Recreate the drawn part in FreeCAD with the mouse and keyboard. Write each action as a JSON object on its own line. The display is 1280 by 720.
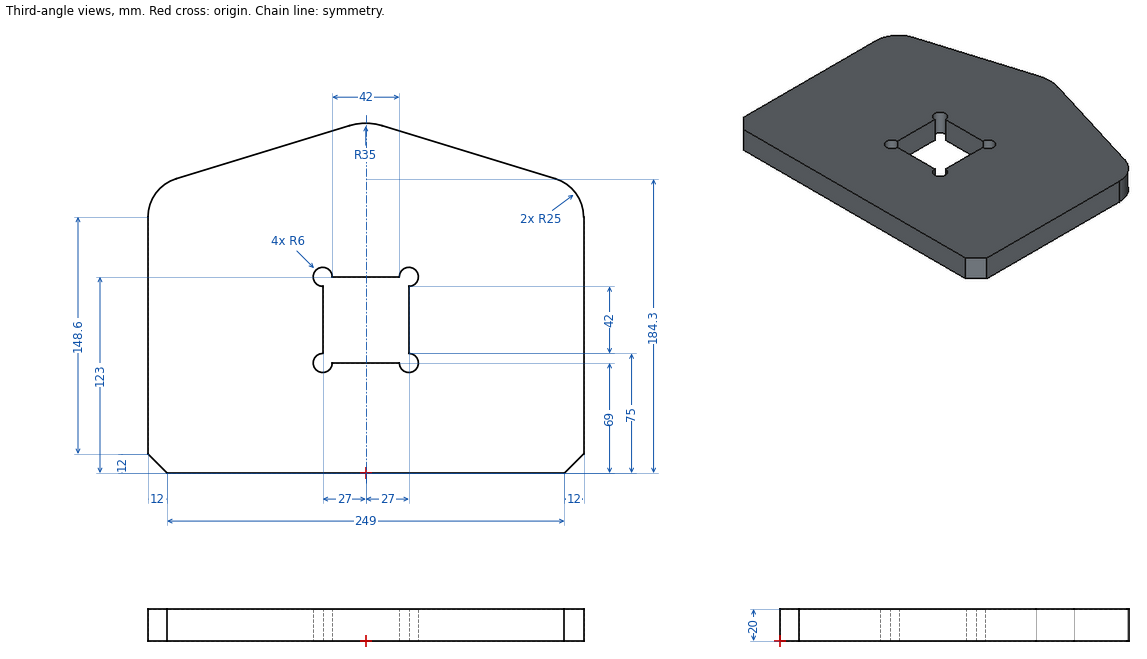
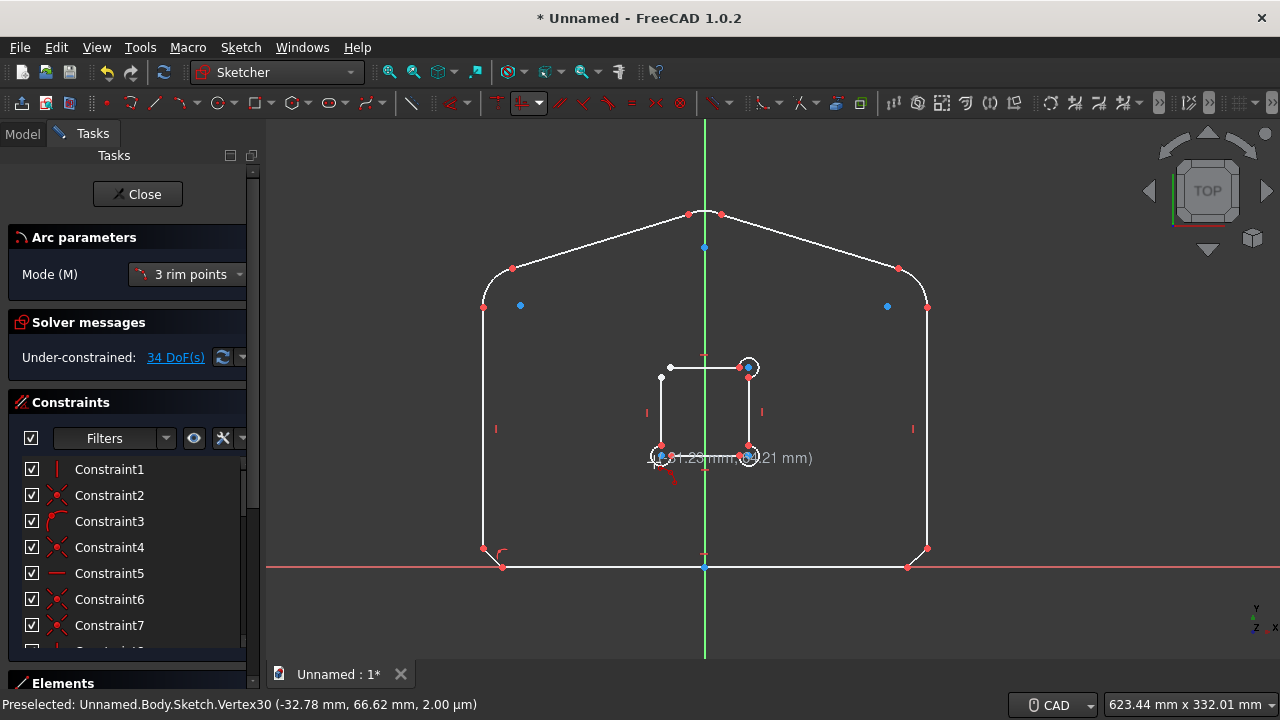
{"action": "left_click", "coordinate": [661, 378]}
{"action": "left_click", "coordinate": [670, 368]}
{"action": "left_click", "coordinate": [654, 360]}
{"action": "key", "text": "Escape"}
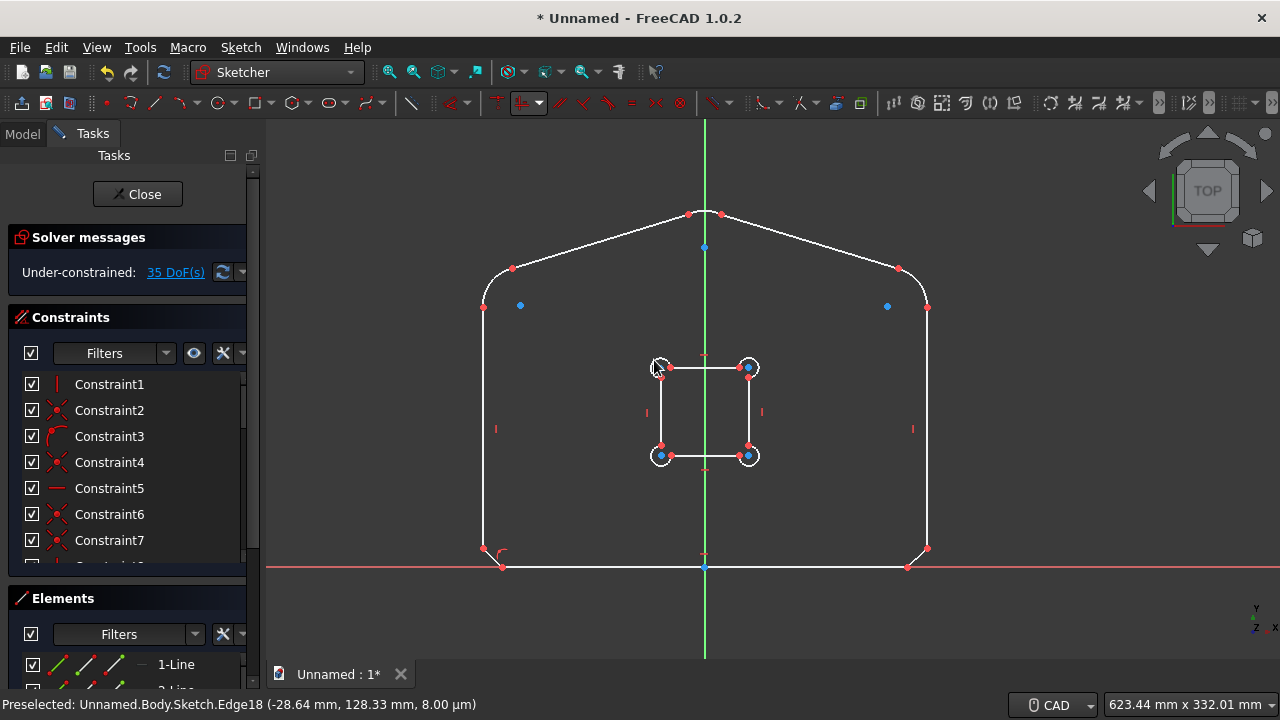
{"action": "left_click", "coordinate": [845, 252]}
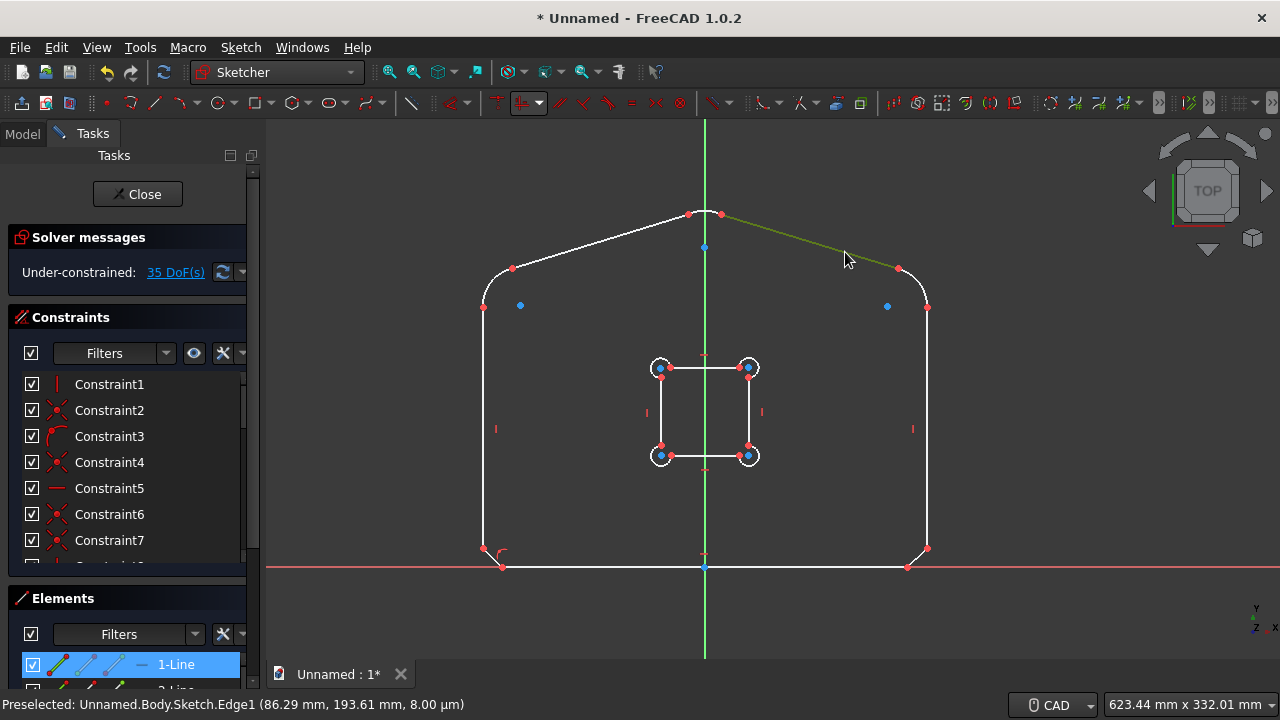
{"action": "left_click", "coordinate": [704, 211]}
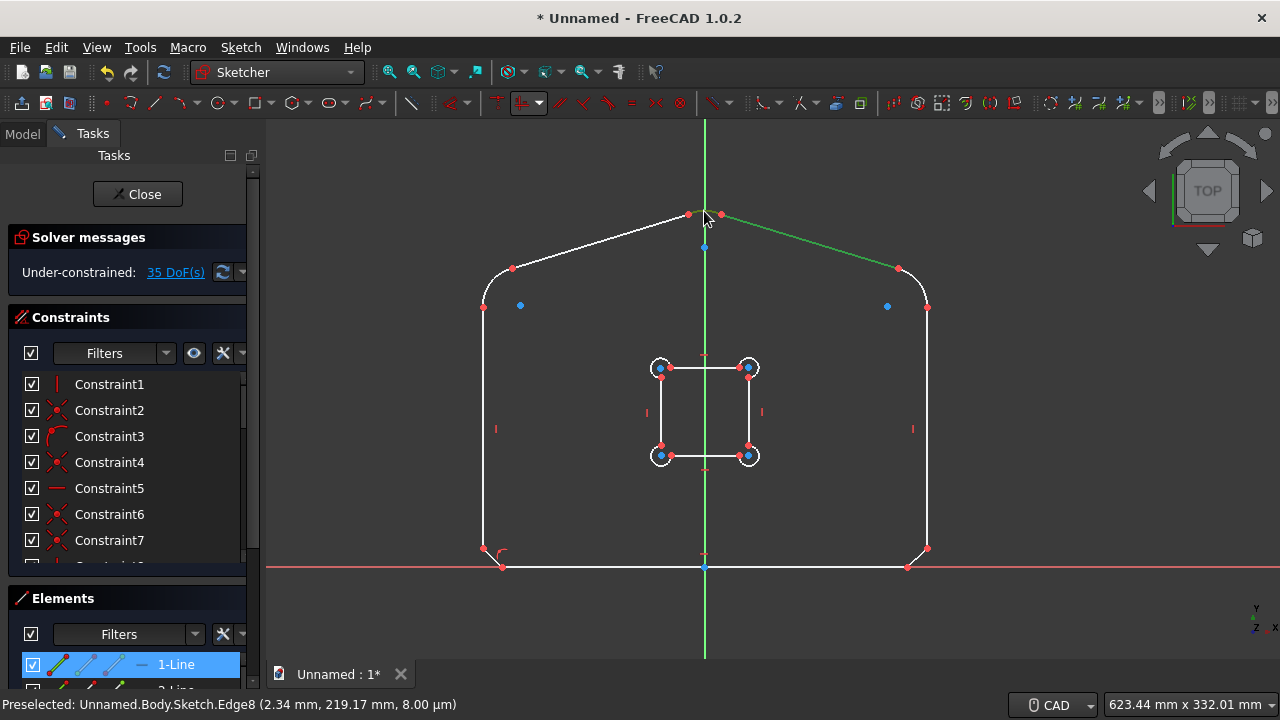
{"action": "left_click", "coordinate": [608, 104]}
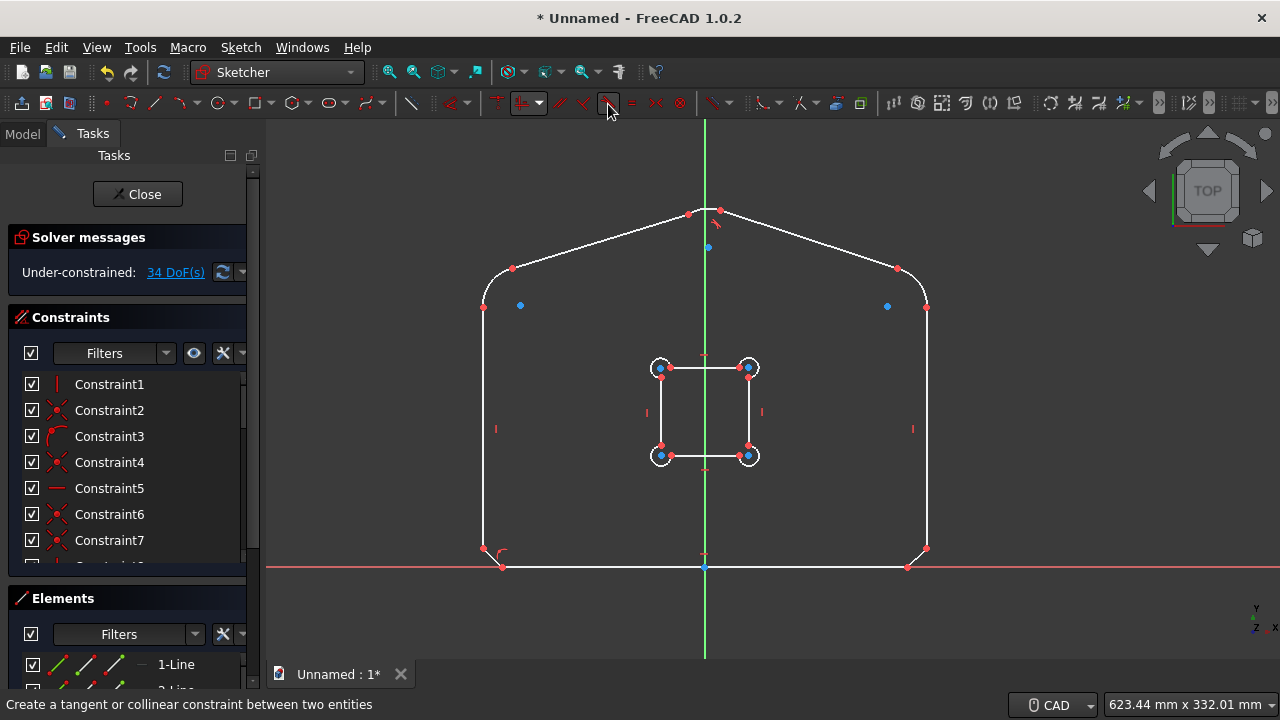
{"action": "left_click", "coordinate": [845, 251]}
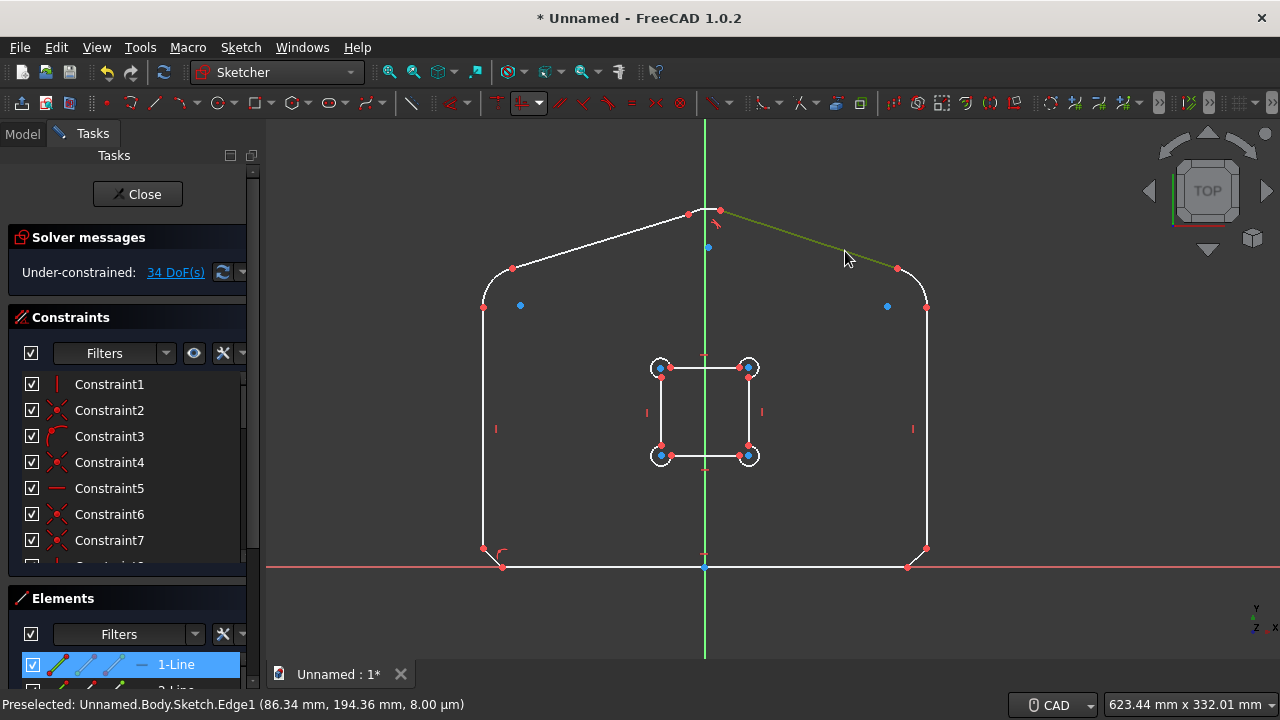
{"action": "left_click", "coordinate": [924, 292]}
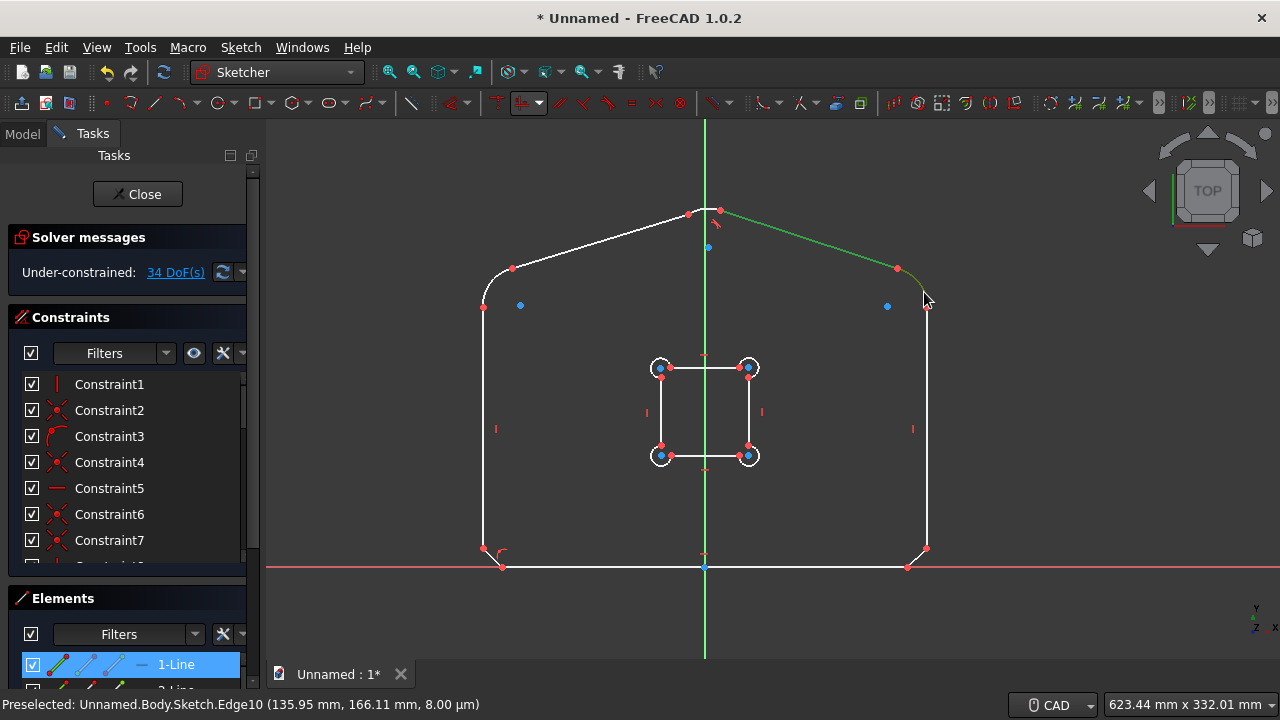
{"action": "left_click", "coordinate": [608, 104]}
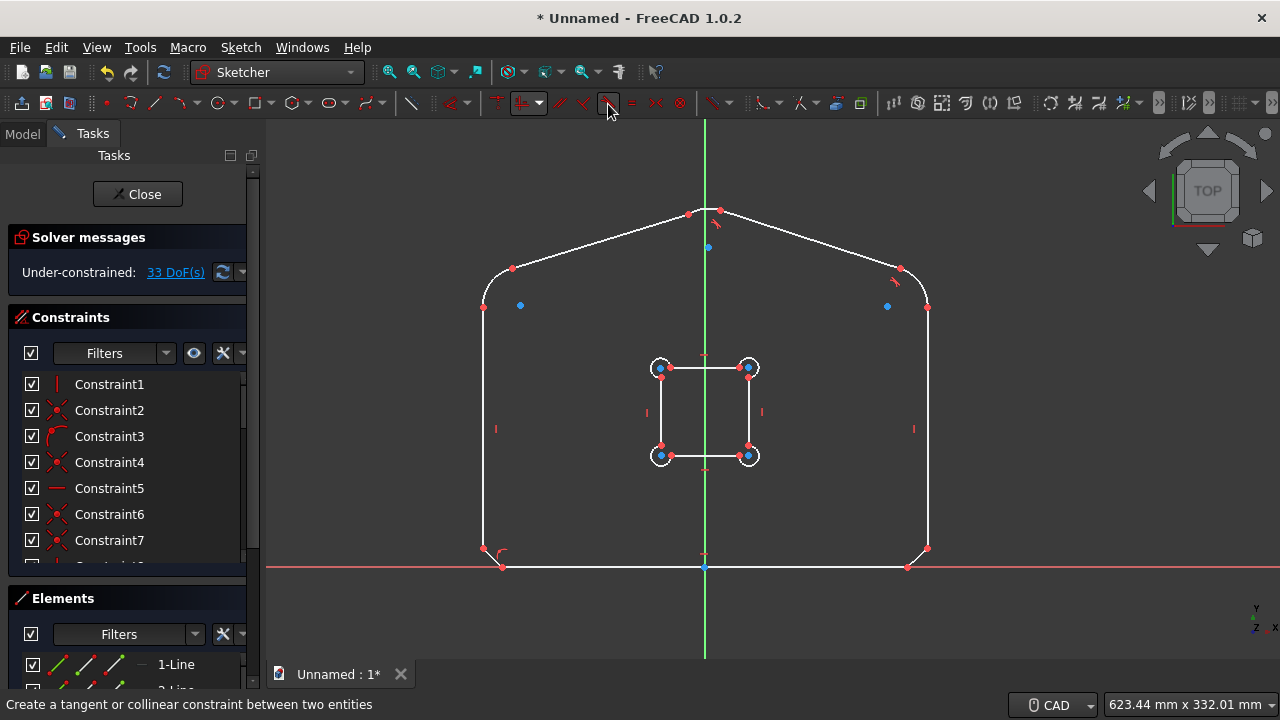
{"action": "left_click", "coordinate": [635, 231]}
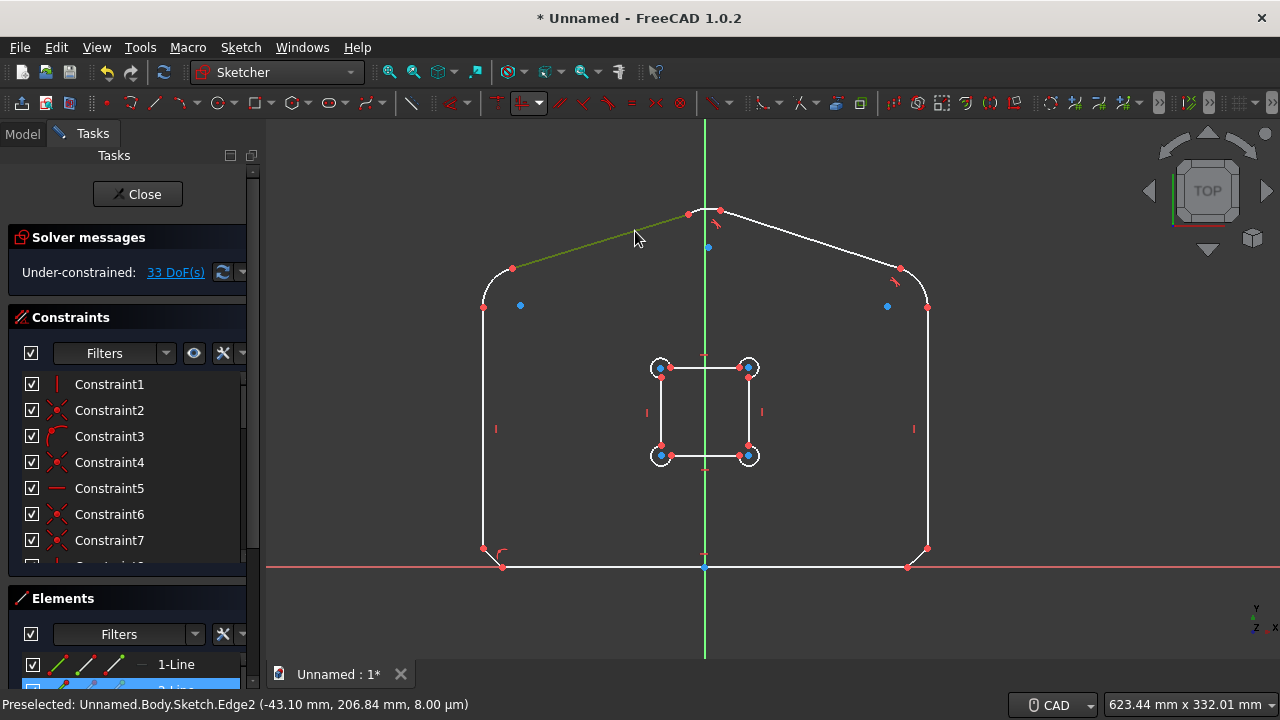
{"action": "left_click", "coordinate": [704, 209]}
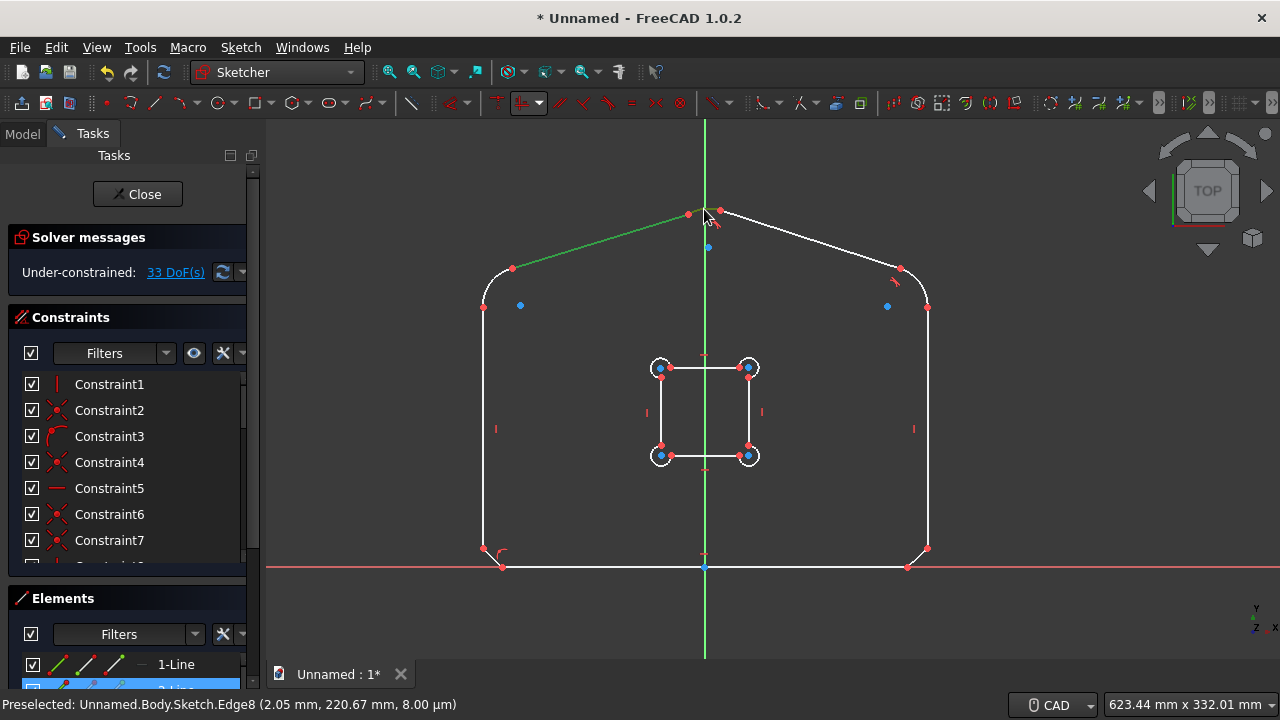
{"action": "left_click", "coordinate": [608, 104]}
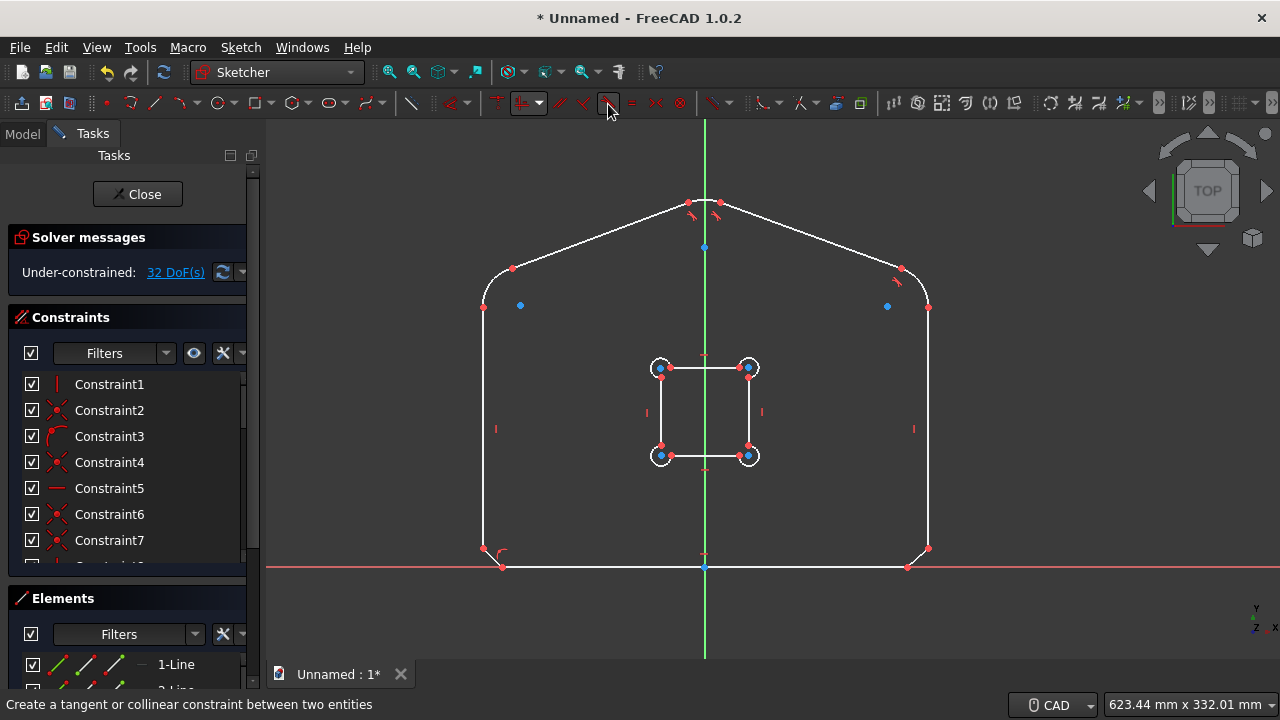
{"action": "left_click", "coordinate": [635, 223]}